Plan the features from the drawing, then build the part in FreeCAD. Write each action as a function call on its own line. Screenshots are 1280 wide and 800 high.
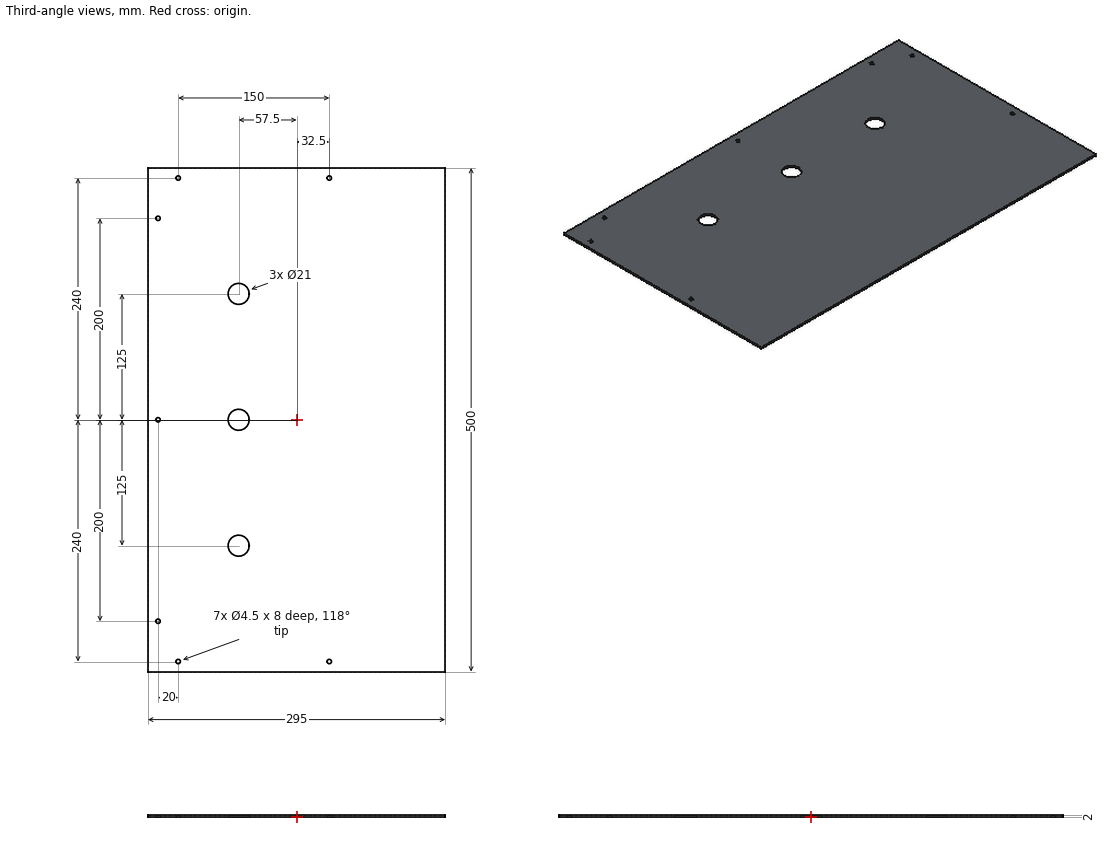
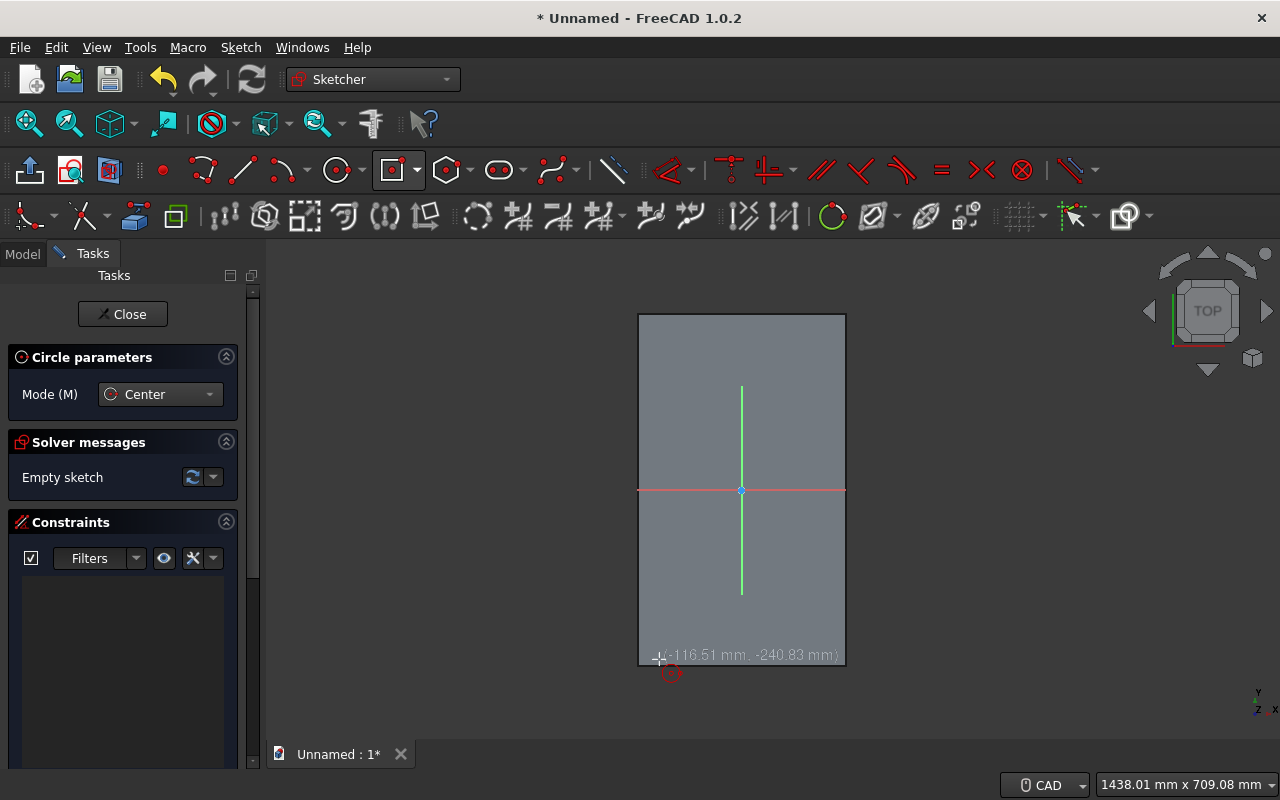
click(659, 659)
move(660, 658)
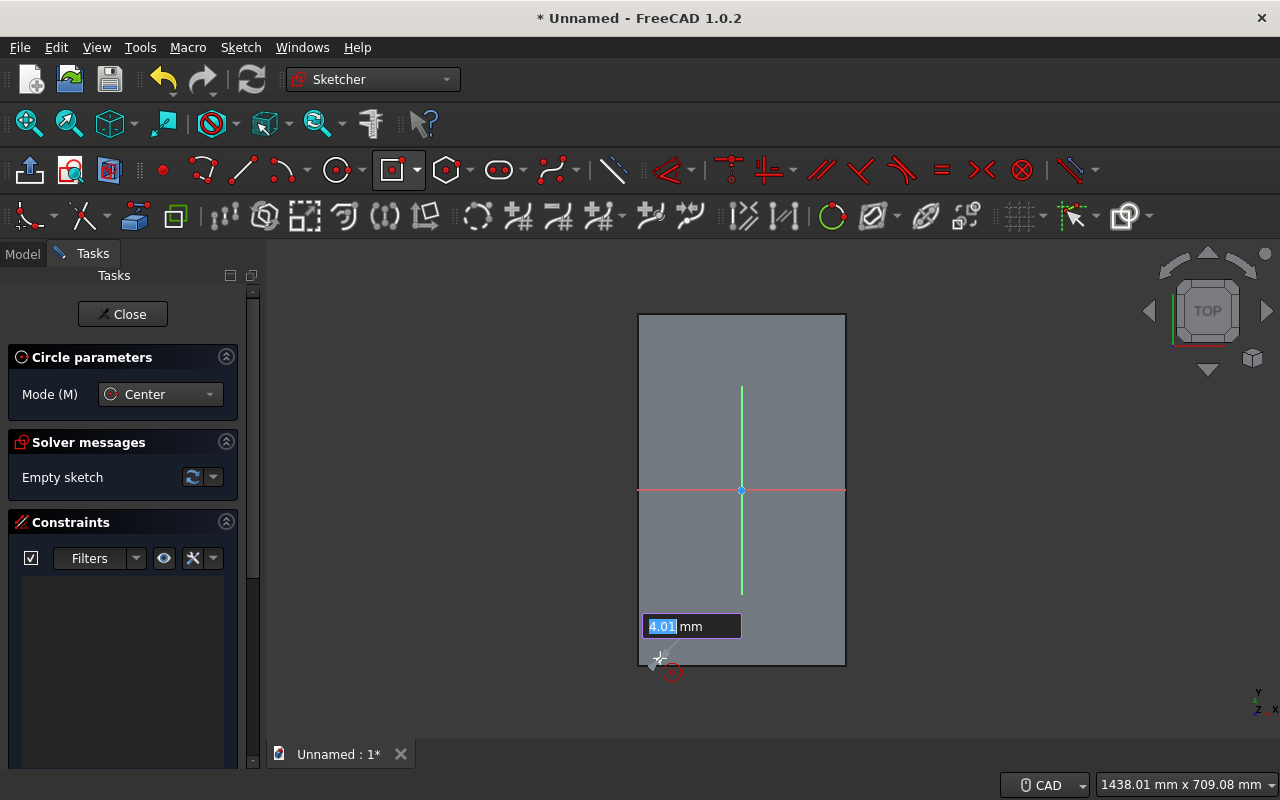
text(4.5)
key(Return)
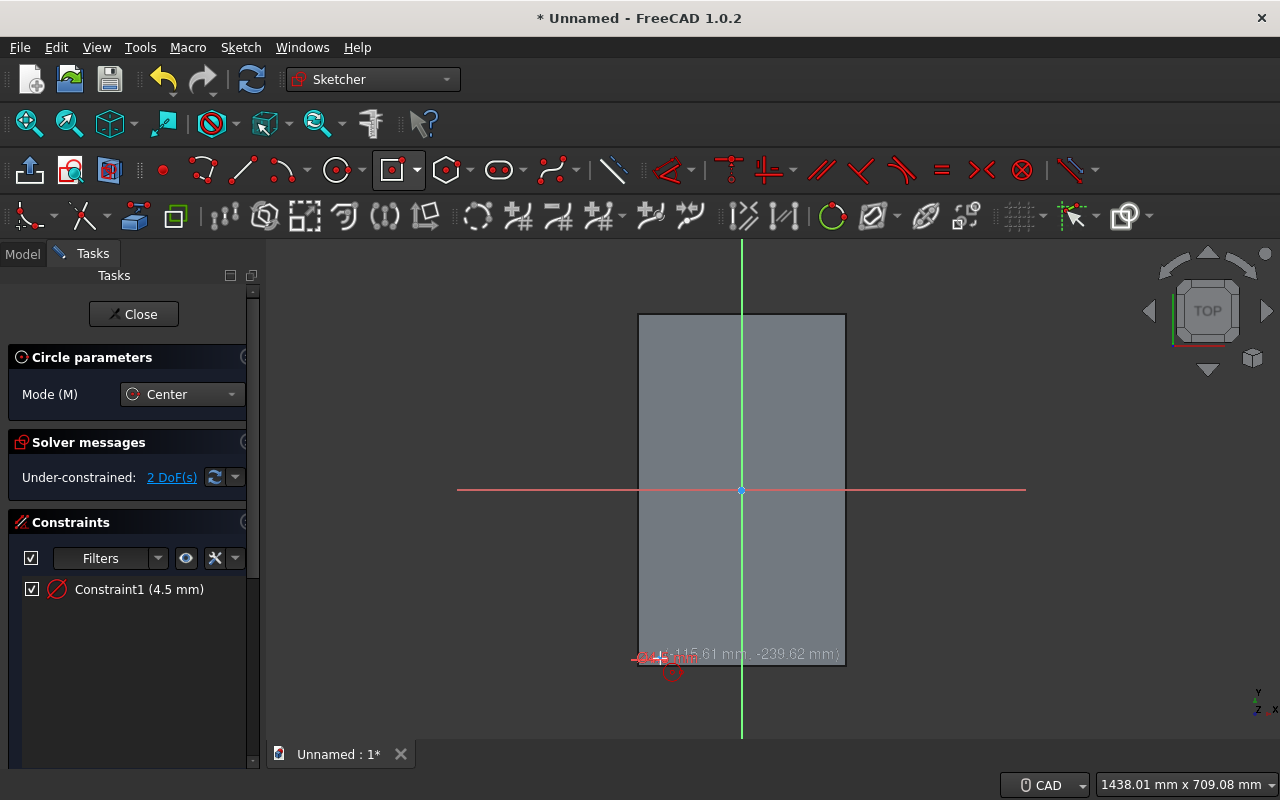
scroll(645, 490, up, 14)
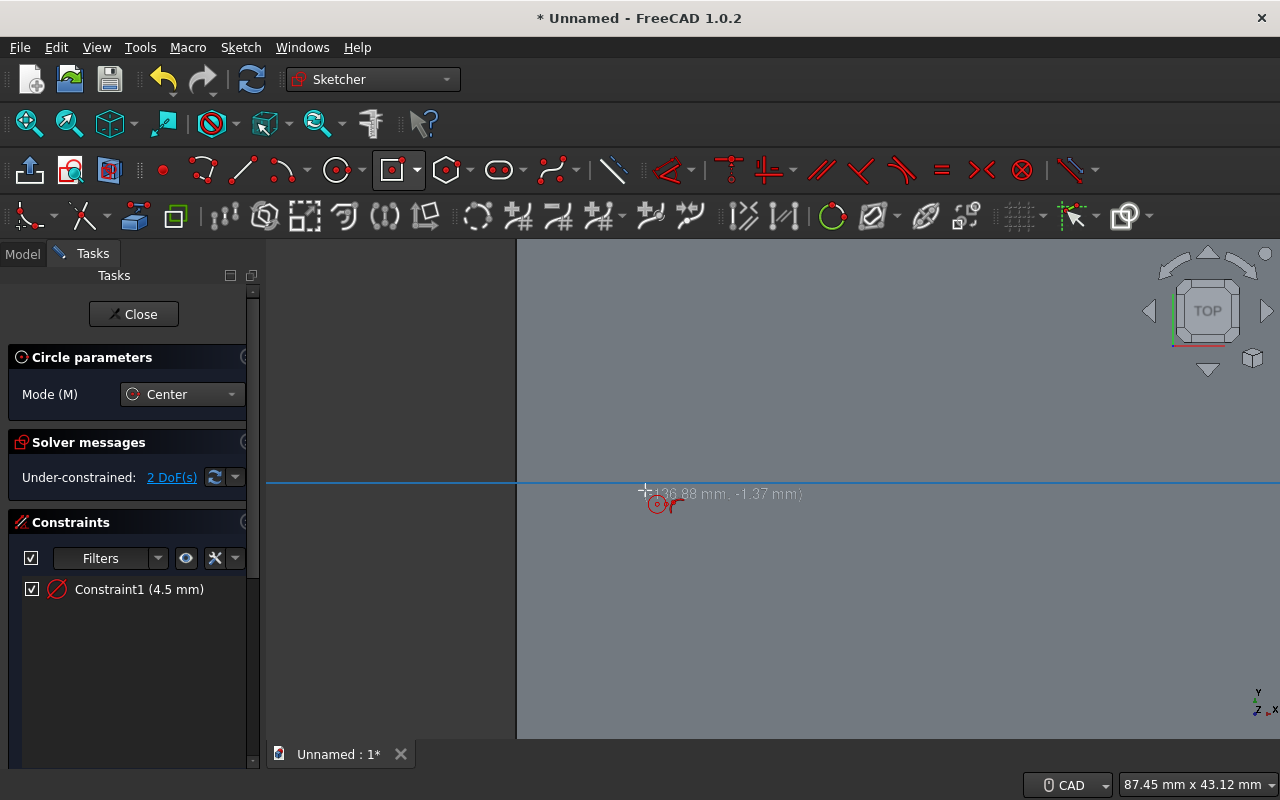
scroll(645, 489, down, 14)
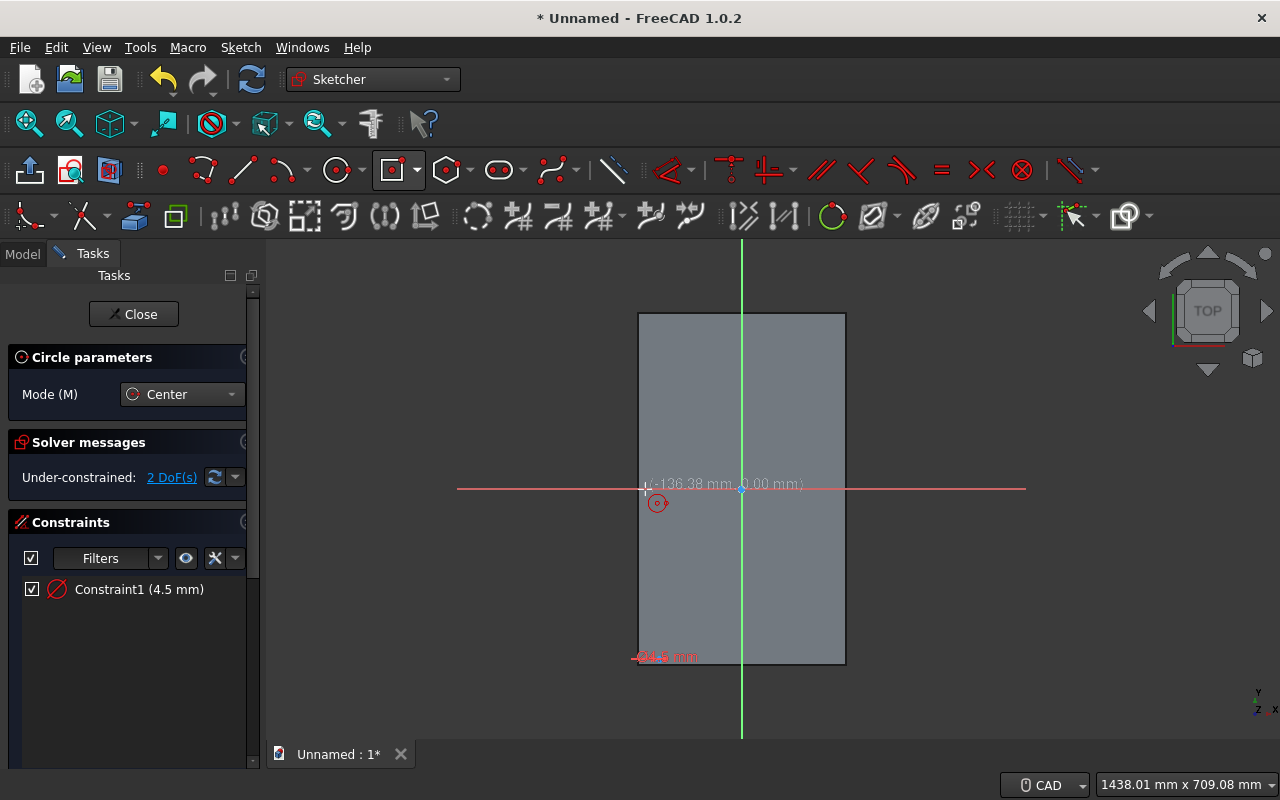
click(645, 489)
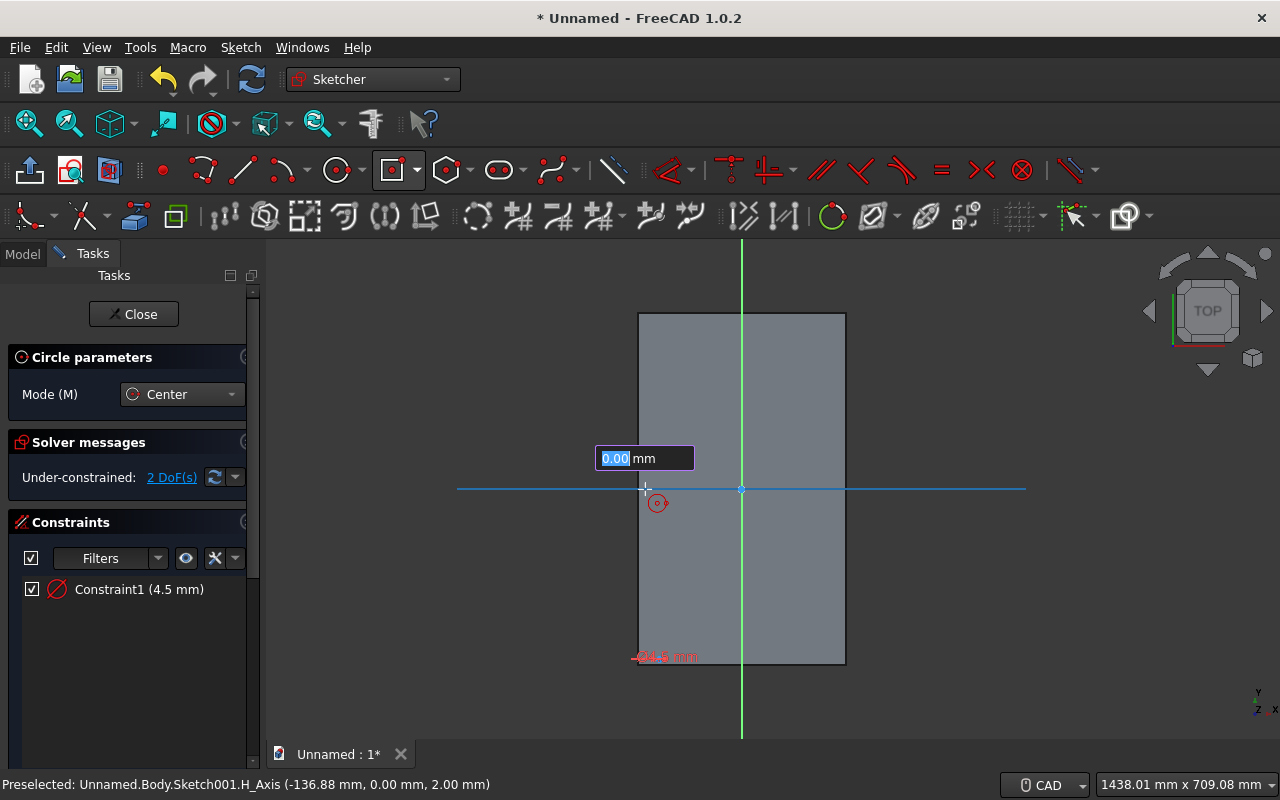
scroll(644, 491, up, 12)
move(640, 481)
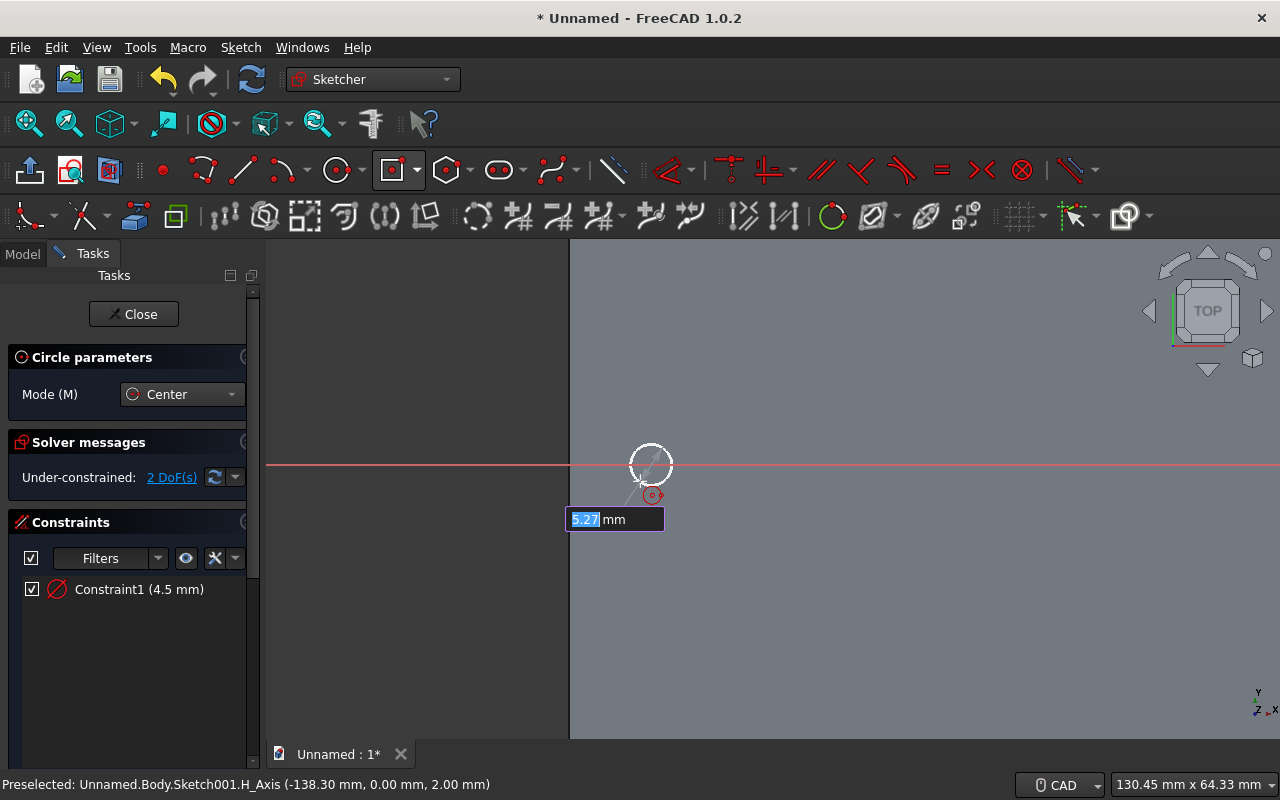
text(4.5)
key(Return)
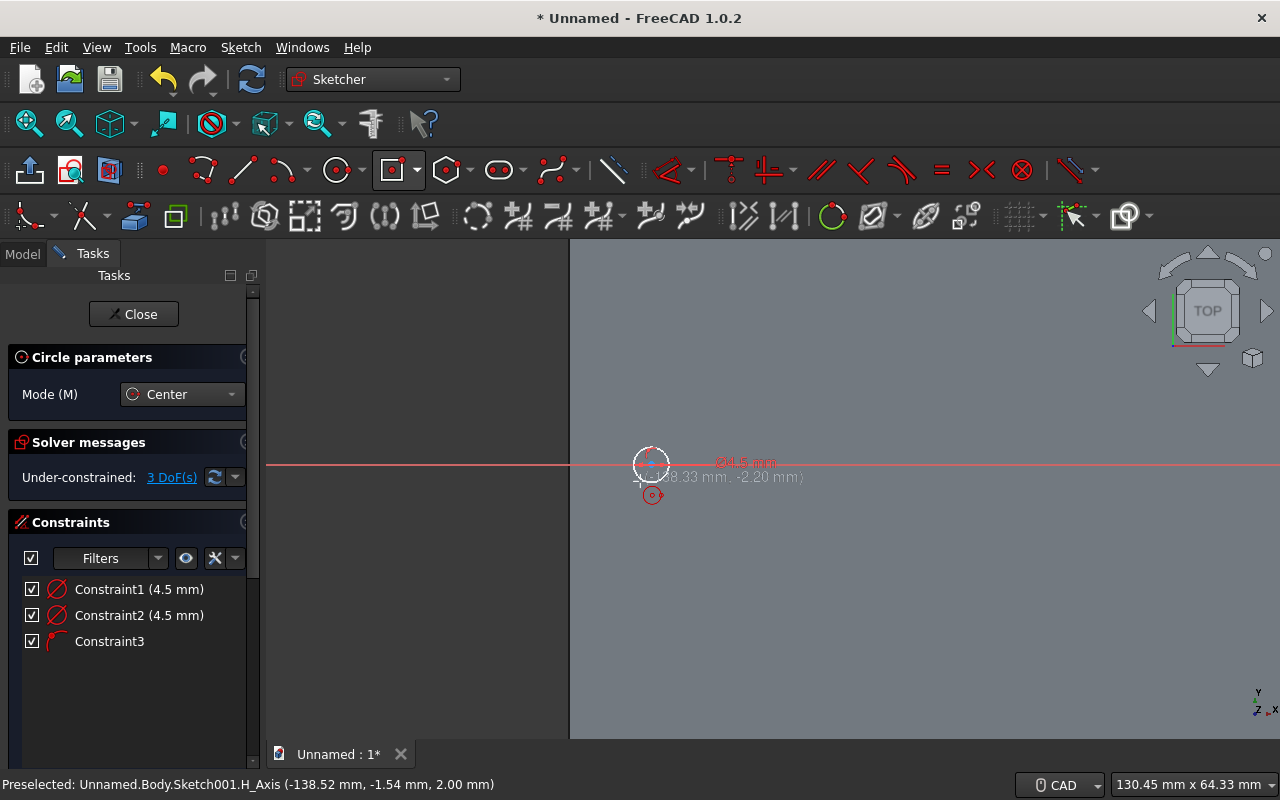
scroll(644, 491, down, 12)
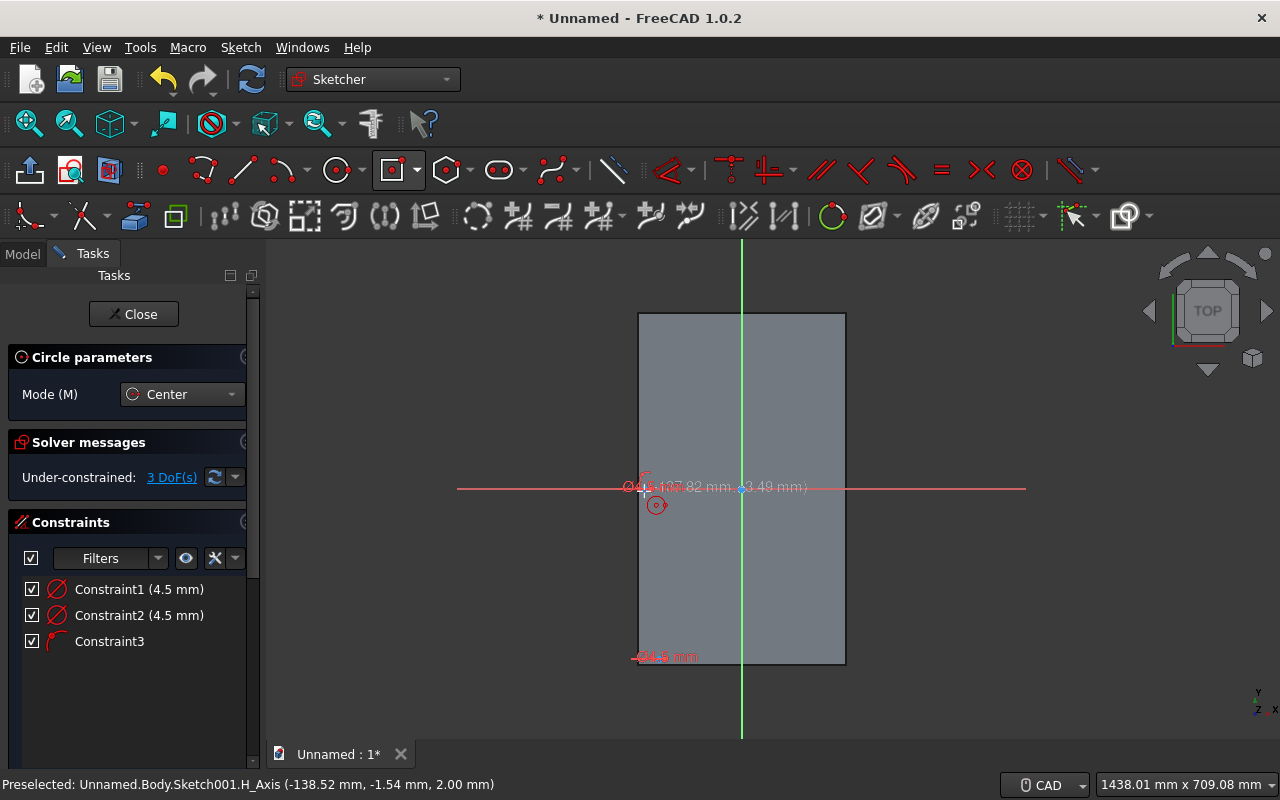
scroll(645, 348, up, 14)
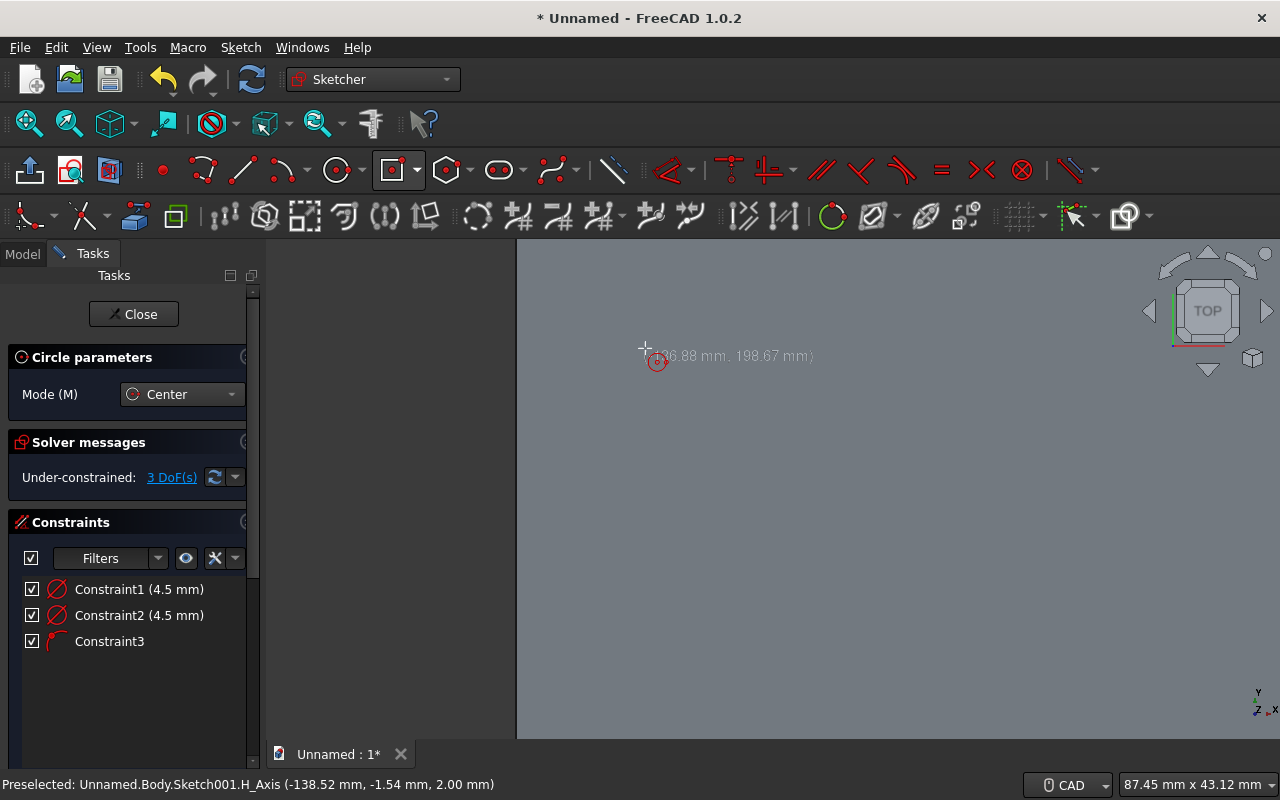
scroll(645, 348, down, 14)